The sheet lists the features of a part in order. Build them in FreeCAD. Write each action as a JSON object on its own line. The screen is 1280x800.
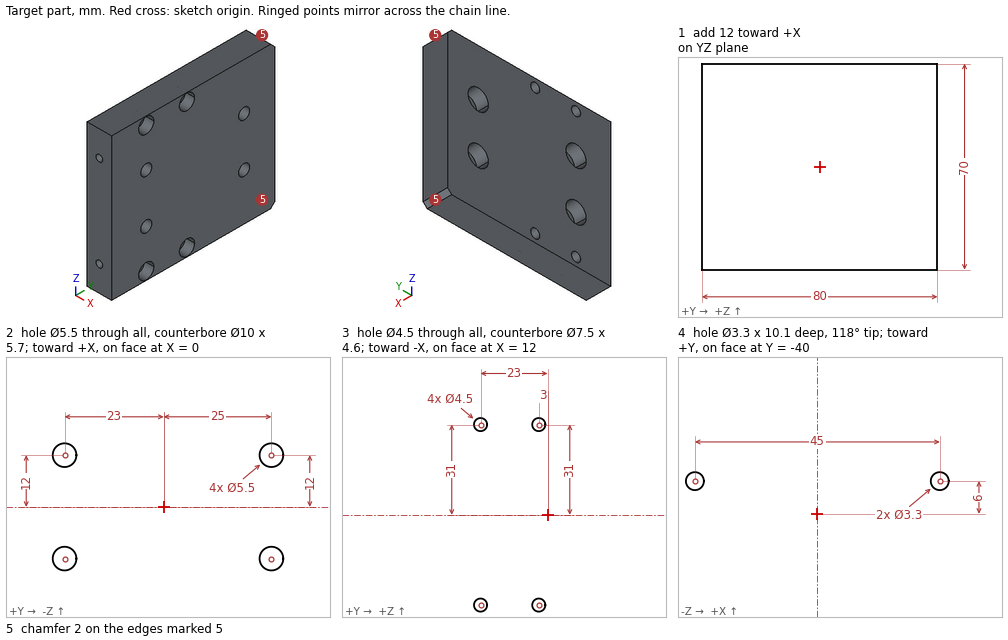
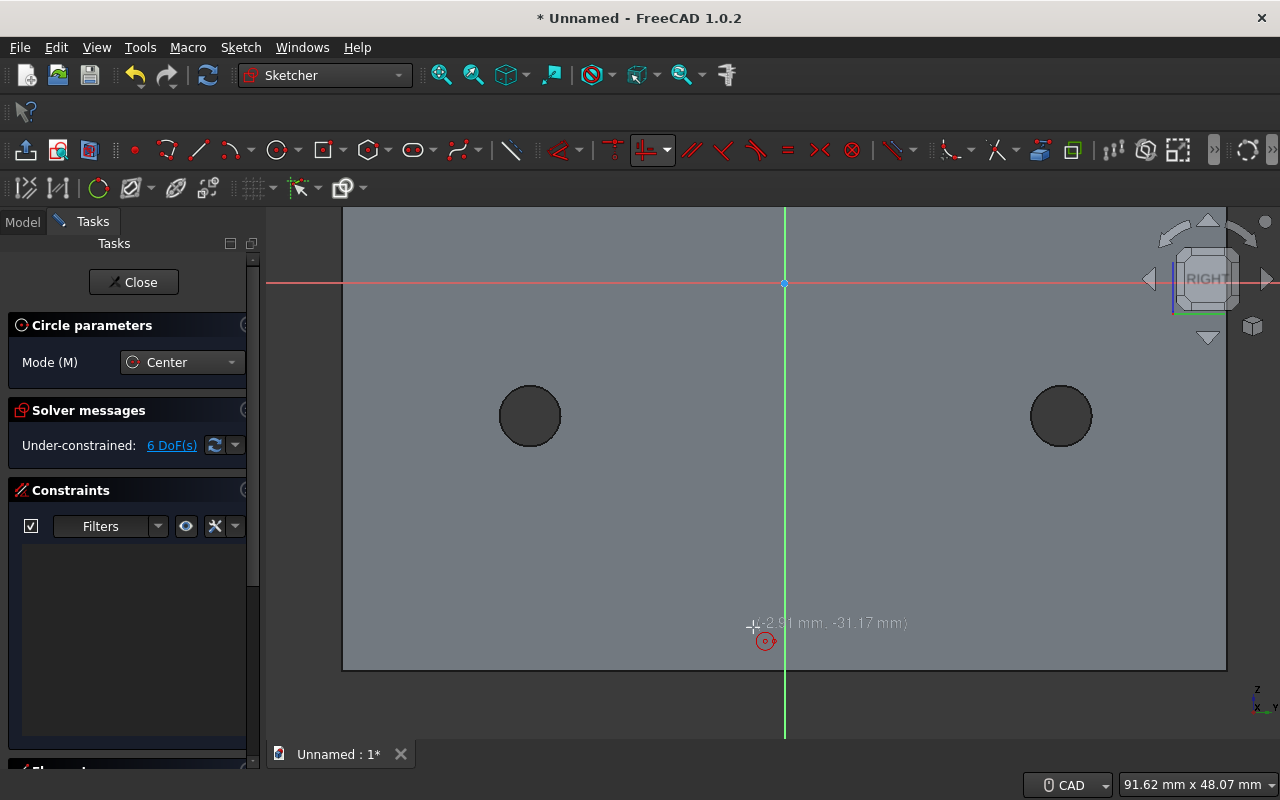
{"action": "left_click", "coordinate": [751, 626]}
{"action": "left_click", "coordinate": [769, 609]}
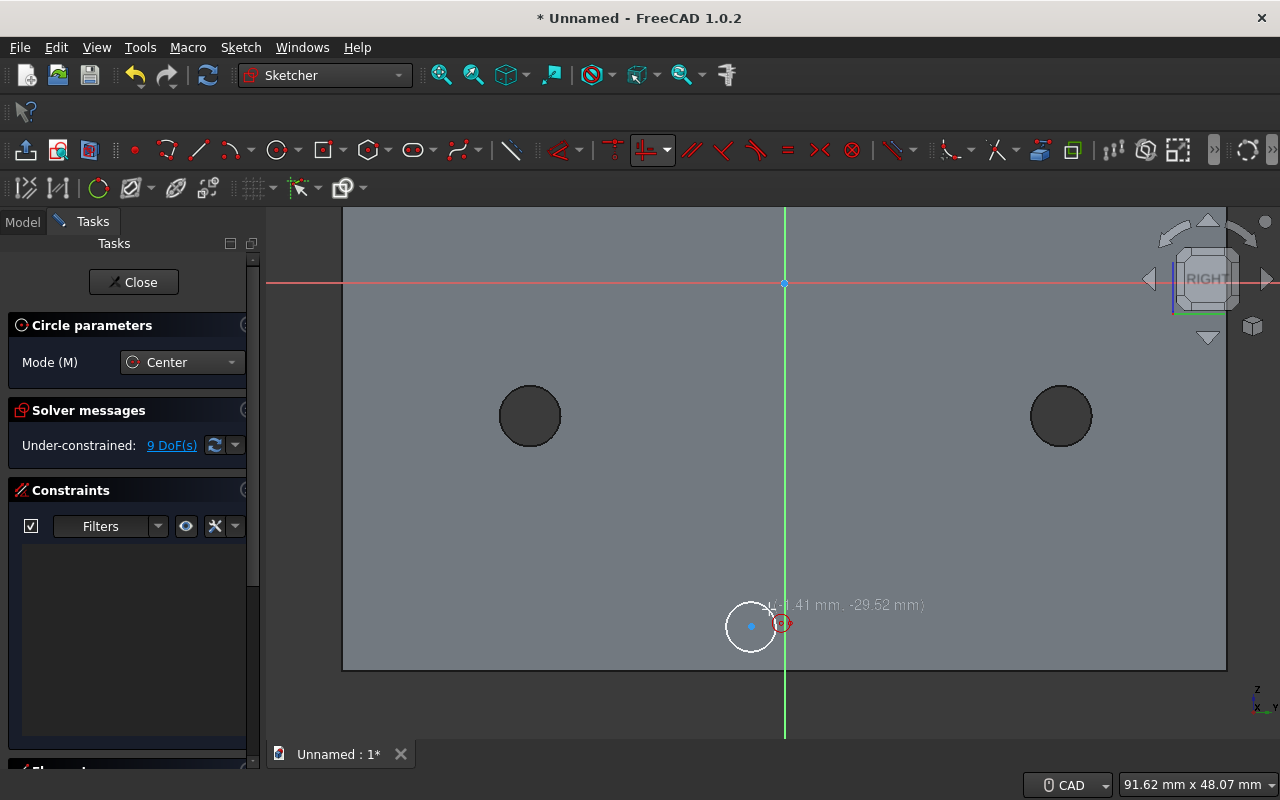
{"action": "left_click", "coordinate": [530, 626]}
{"action": "left_click", "coordinate": [548, 609]}
{"action": "key", "text": "Escape"}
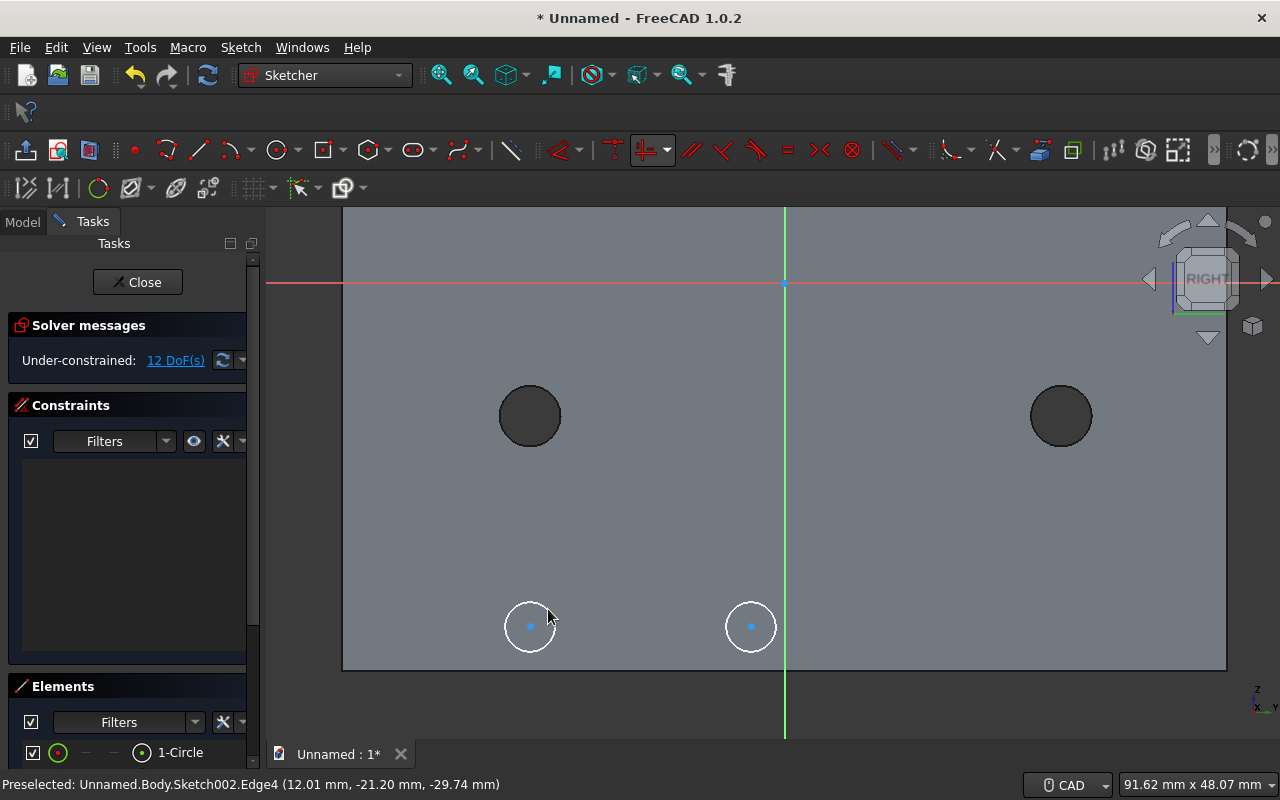
{"action": "scroll", "coordinate": [753, 628], "scroll_direction": "down", "scroll_amount": 4}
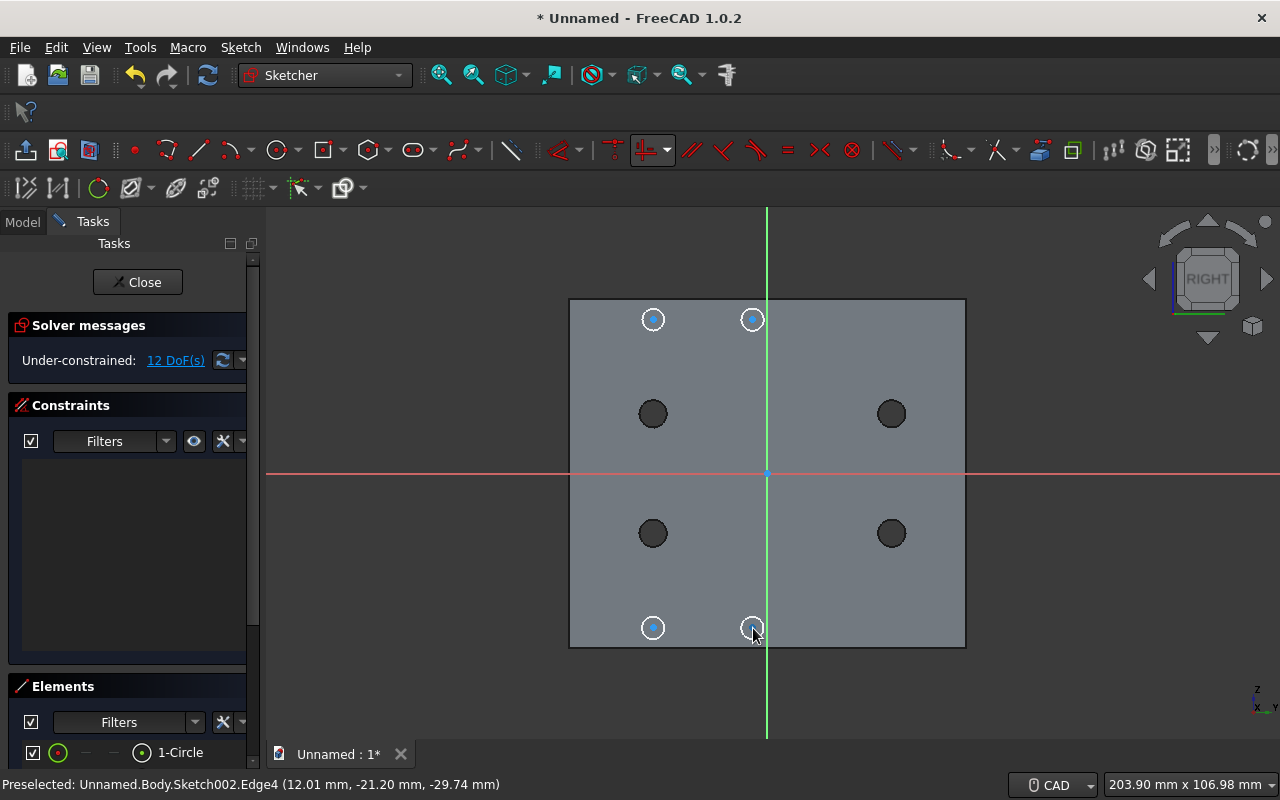
{"action": "scroll", "coordinate": [661, 312], "scroll_direction": "up", "scroll_amount": 2}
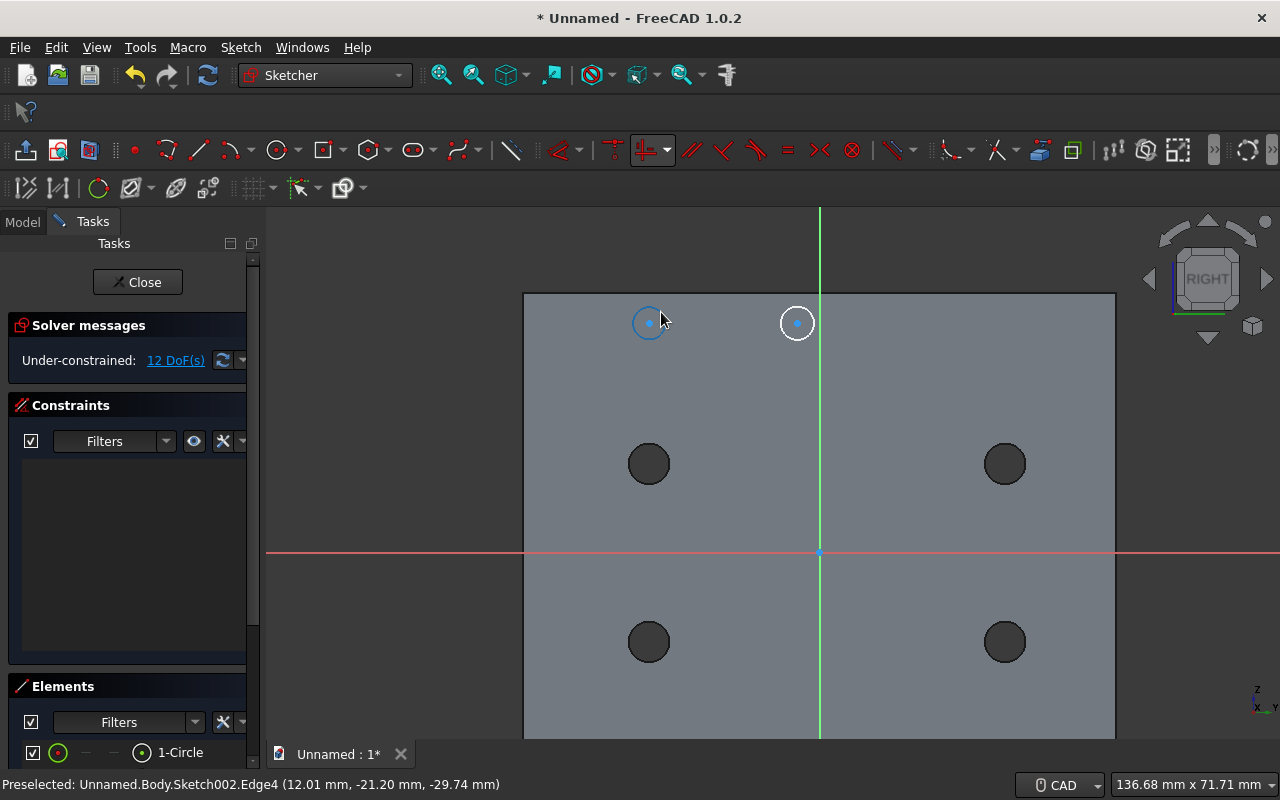
{"action": "left_click", "coordinate": [661, 312]}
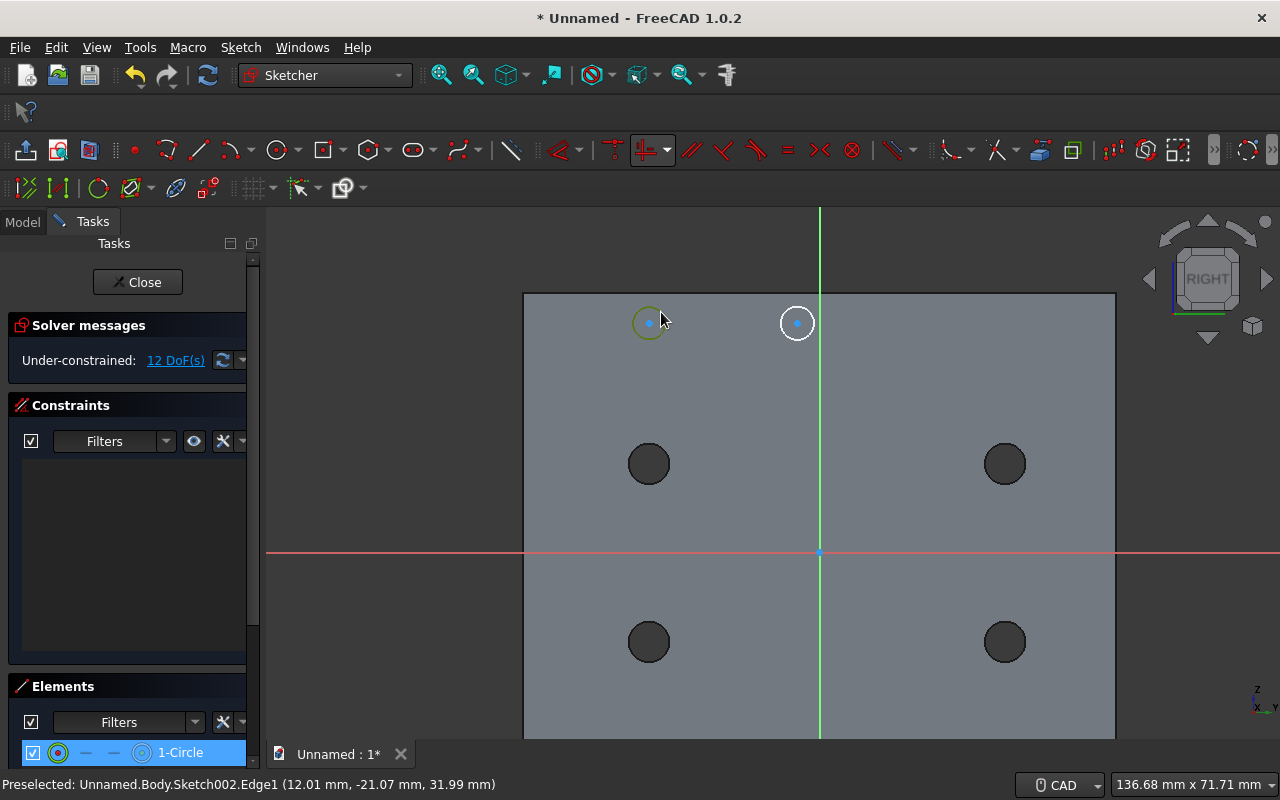
{"action": "scroll", "coordinate": [809, 312], "scroll_direction": "up", "scroll_amount": 2}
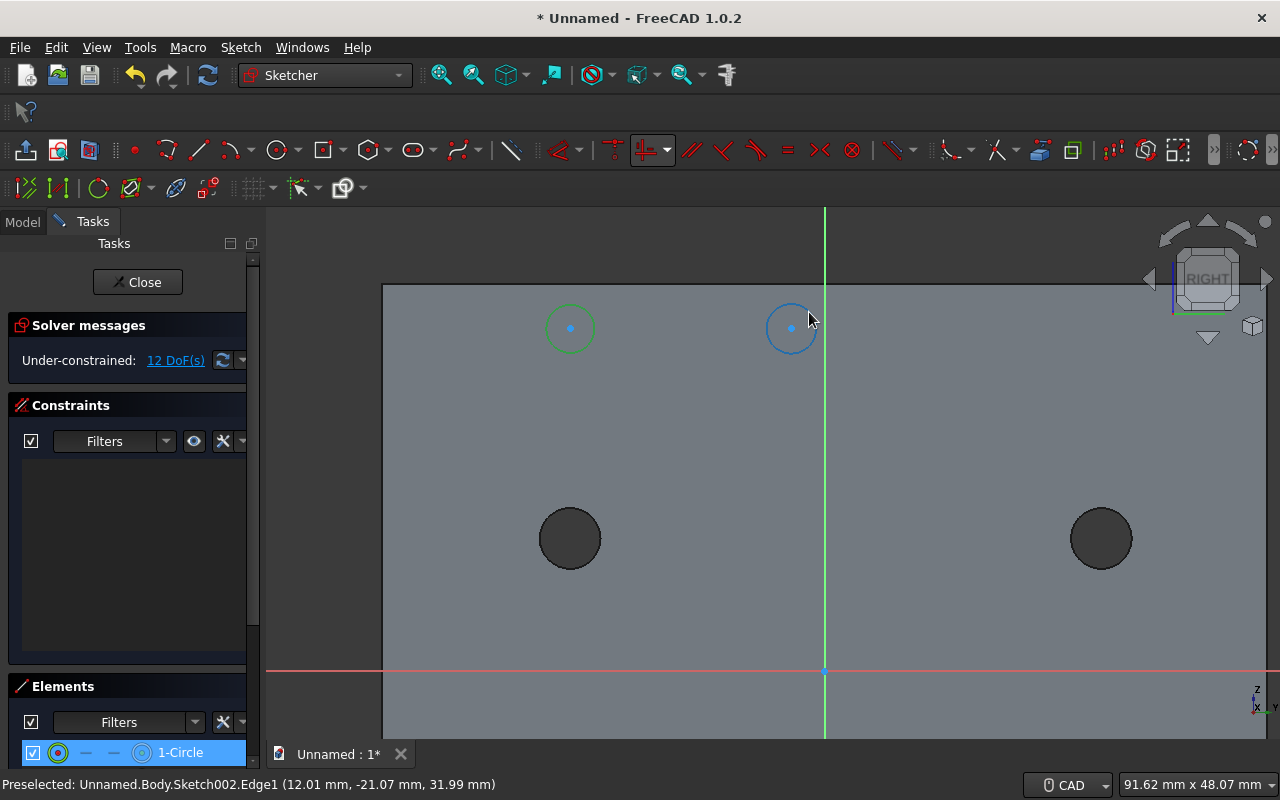
{"action": "left_click", "coordinate": [809, 311]}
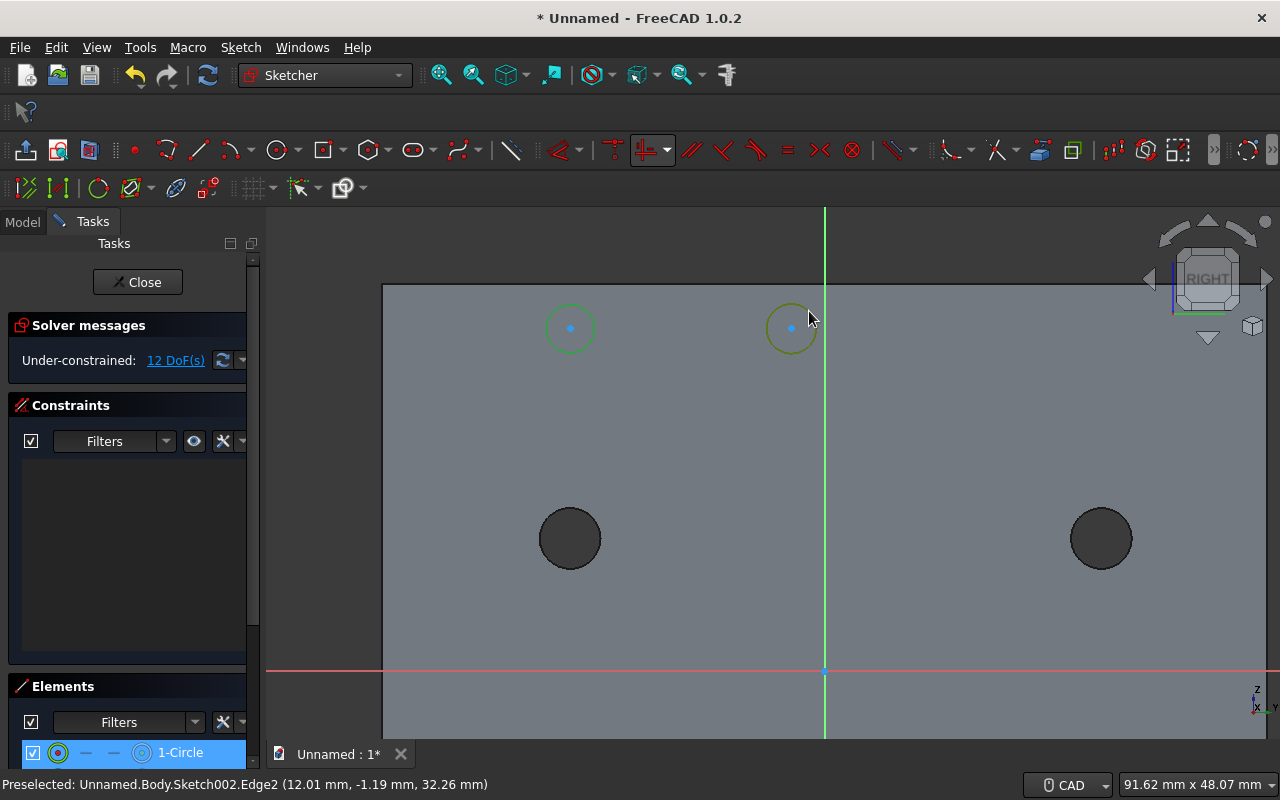
{"action": "scroll", "coordinate": [720, 311], "scroll_direction": "down", "scroll_amount": 4}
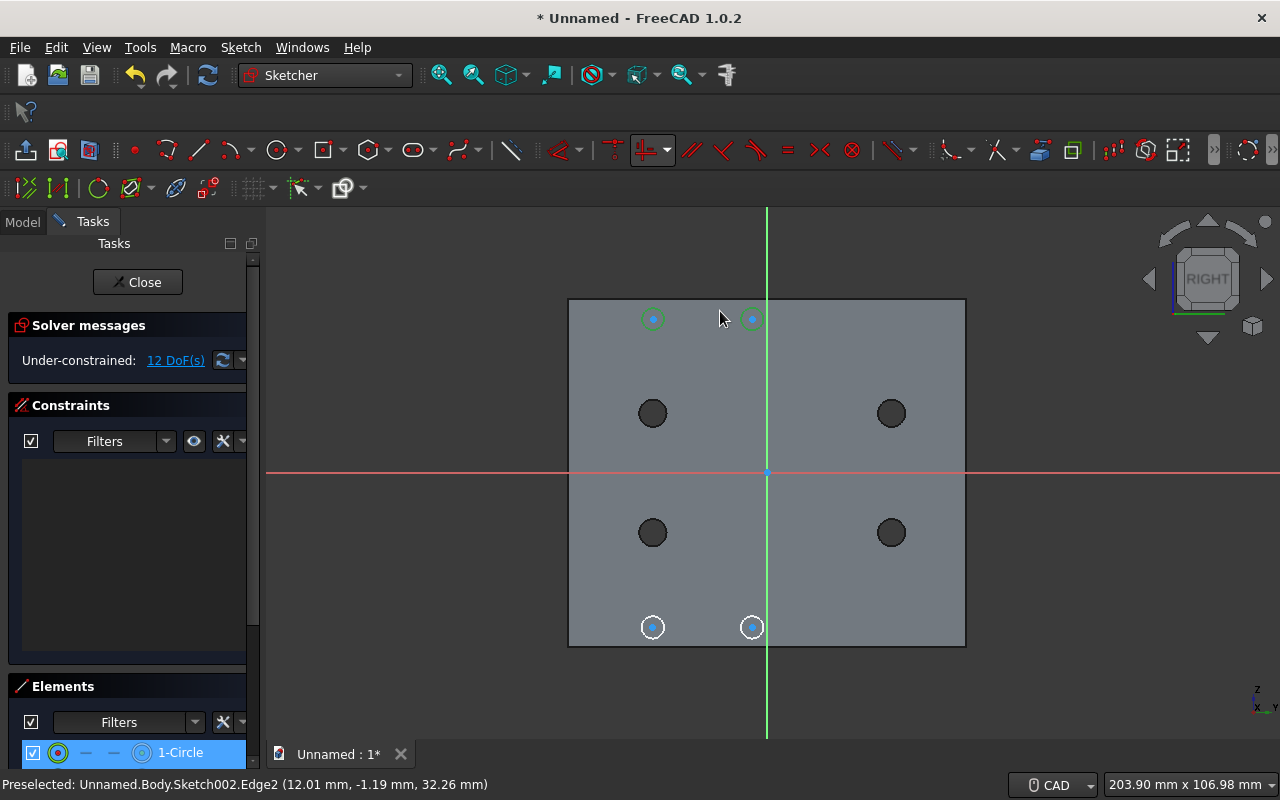
{"action": "scroll", "coordinate": [760, 620], "scroll_direction": "up", "scroll_amount": 4}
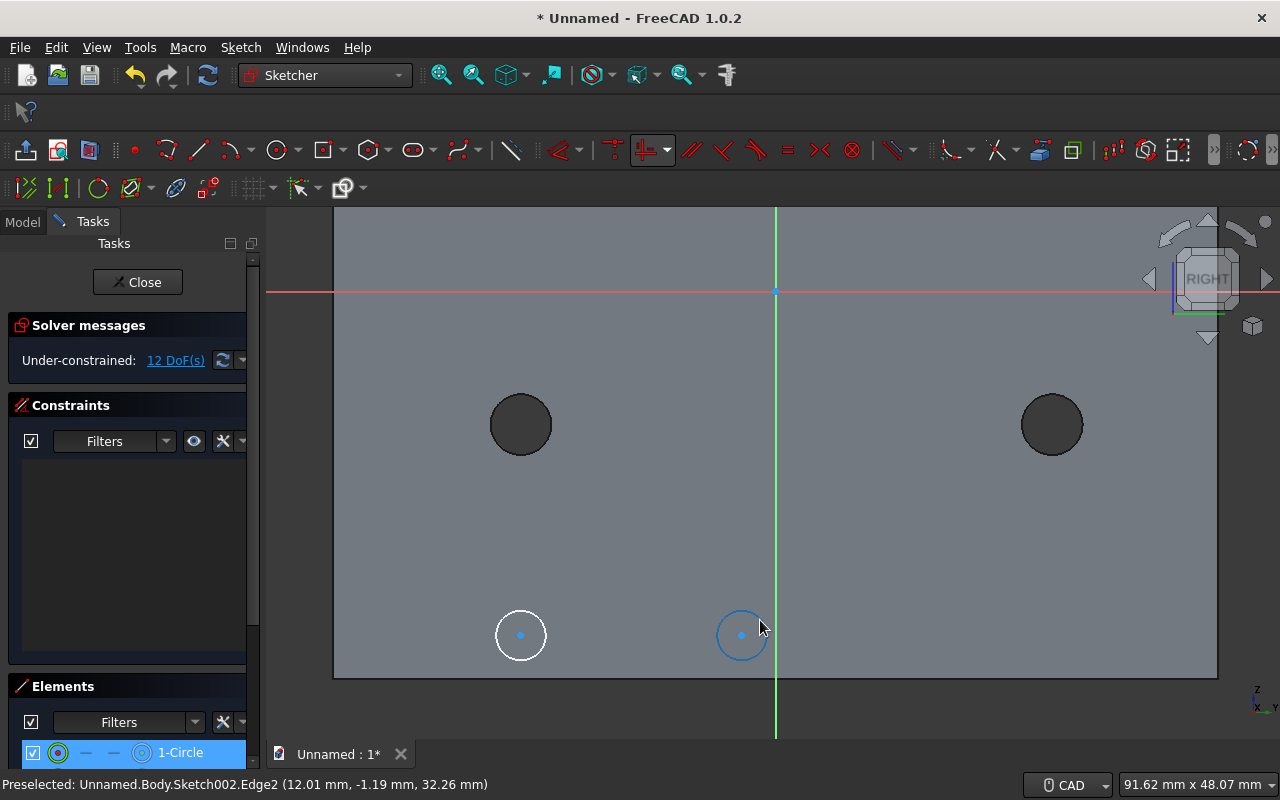
{"action": "left_click", "coordinate": [759, 618]}